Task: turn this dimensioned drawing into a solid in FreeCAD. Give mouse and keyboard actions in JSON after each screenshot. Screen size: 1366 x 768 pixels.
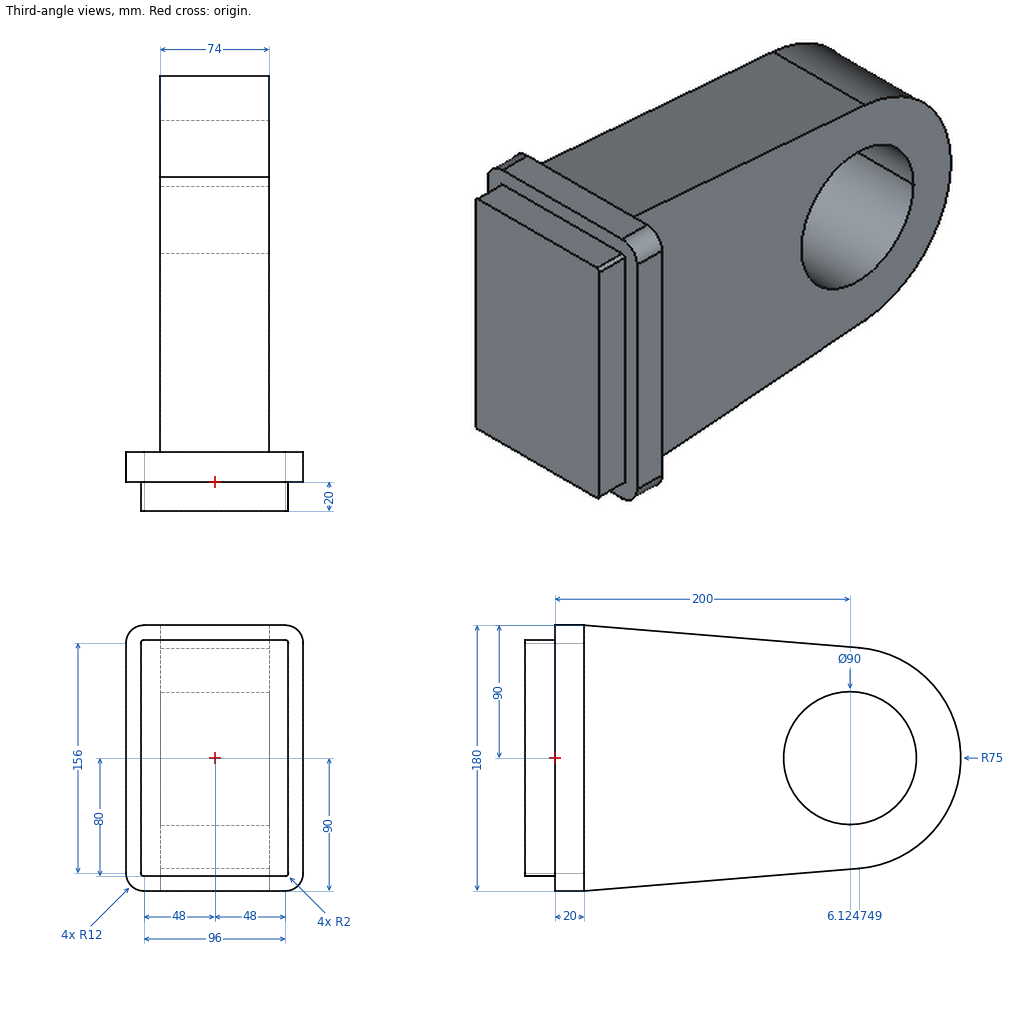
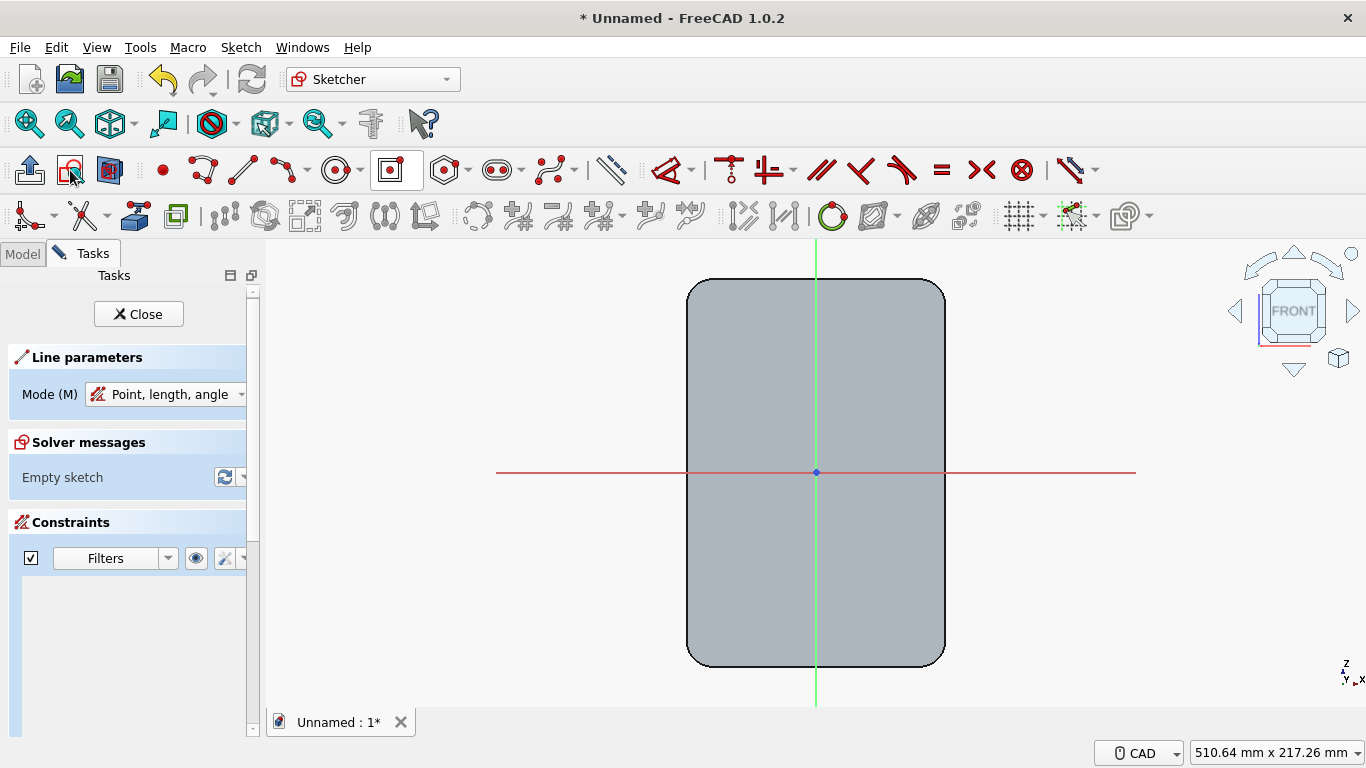
{"action": "left_click", "coordinate": [713, 645]}
{"action": "left_click", "coordinate": [919, 645]}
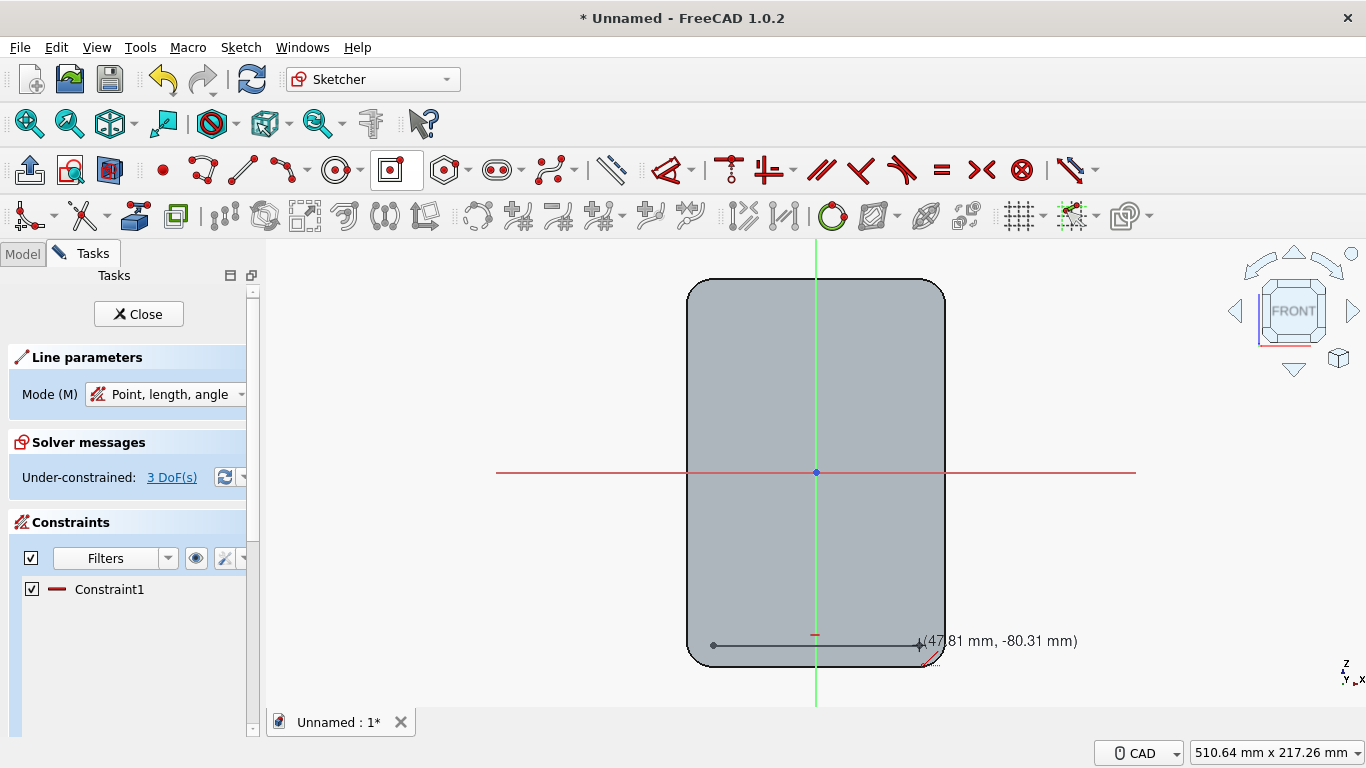
{"action": "scroll", "coordinate": [924, 641], "scroll_direction": "up", "scroll_amount": 5}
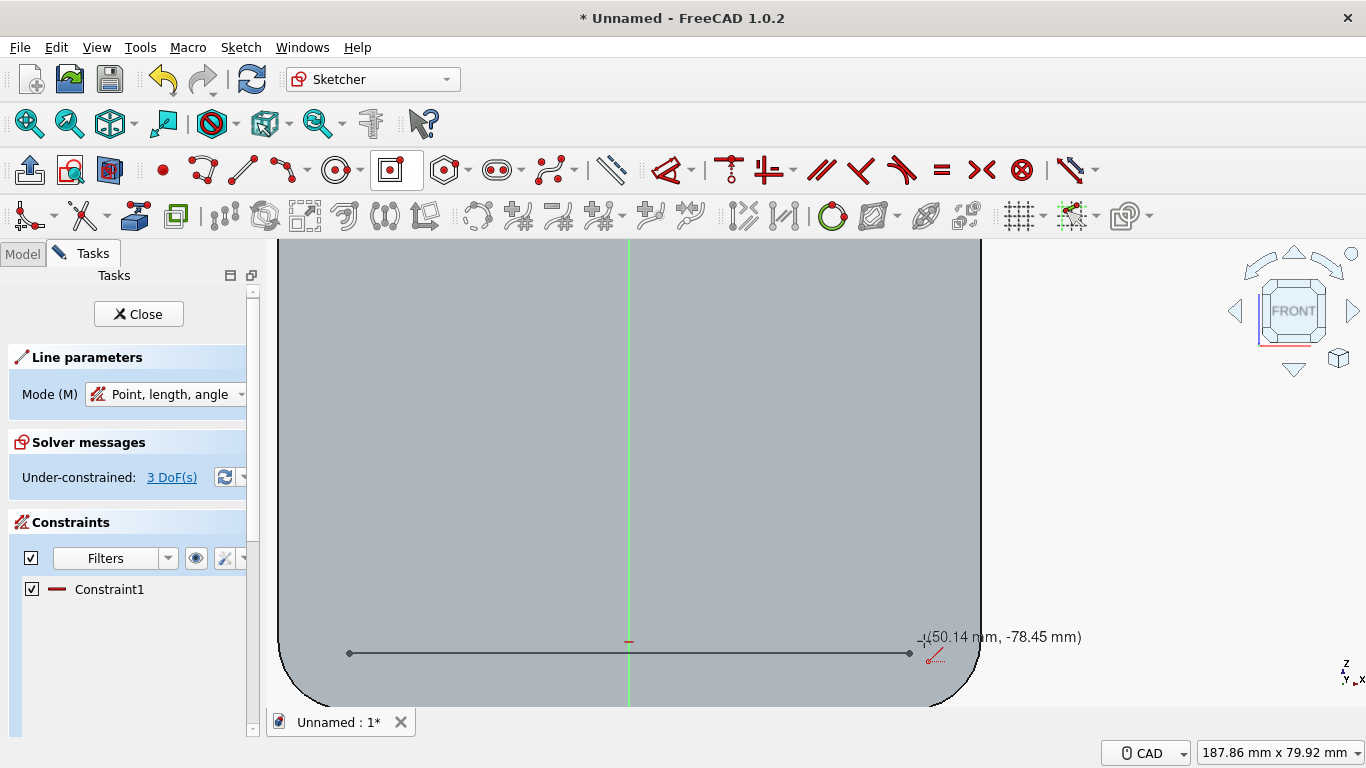
{"action": "left_click", "coordinate": [922, 640]}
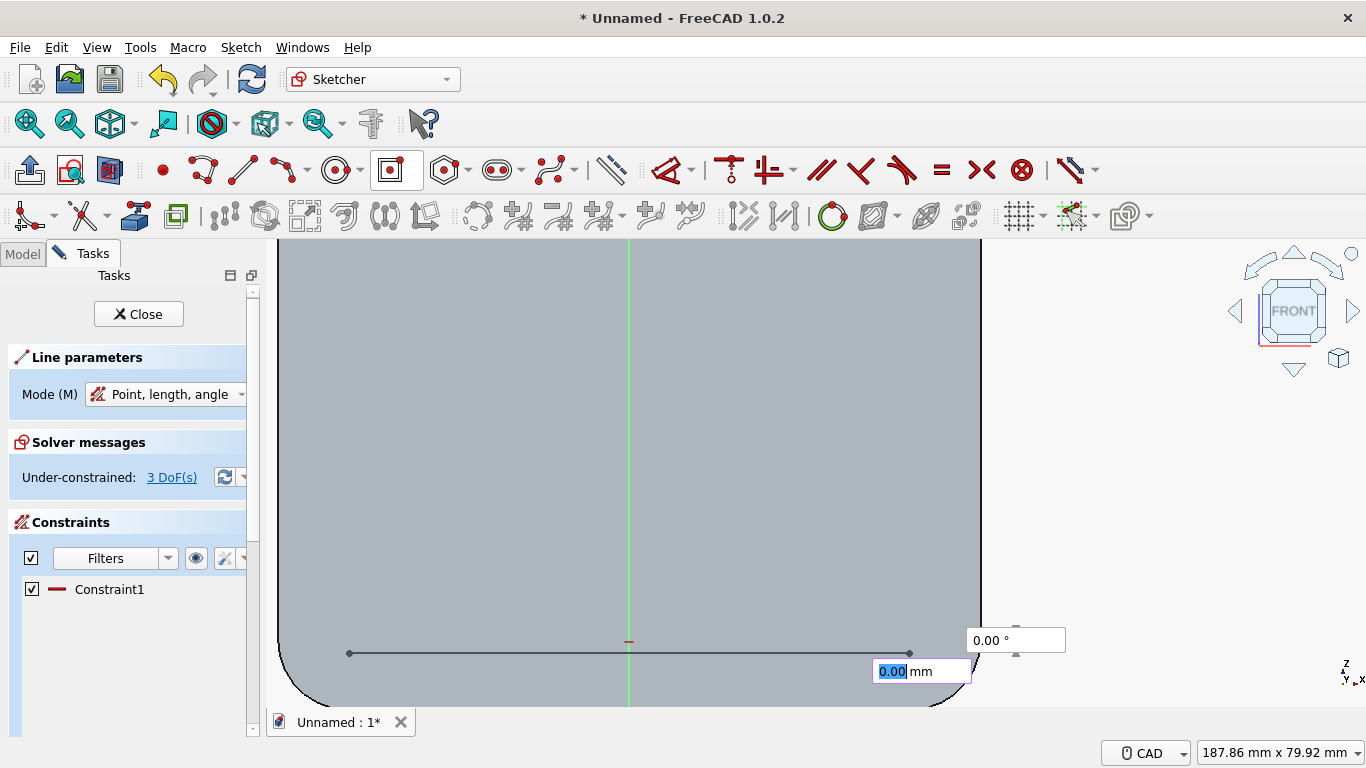
{"action": "scroll", "coordinate": [798, 598], "scroll_direction": "down", "scroll_amount": 6}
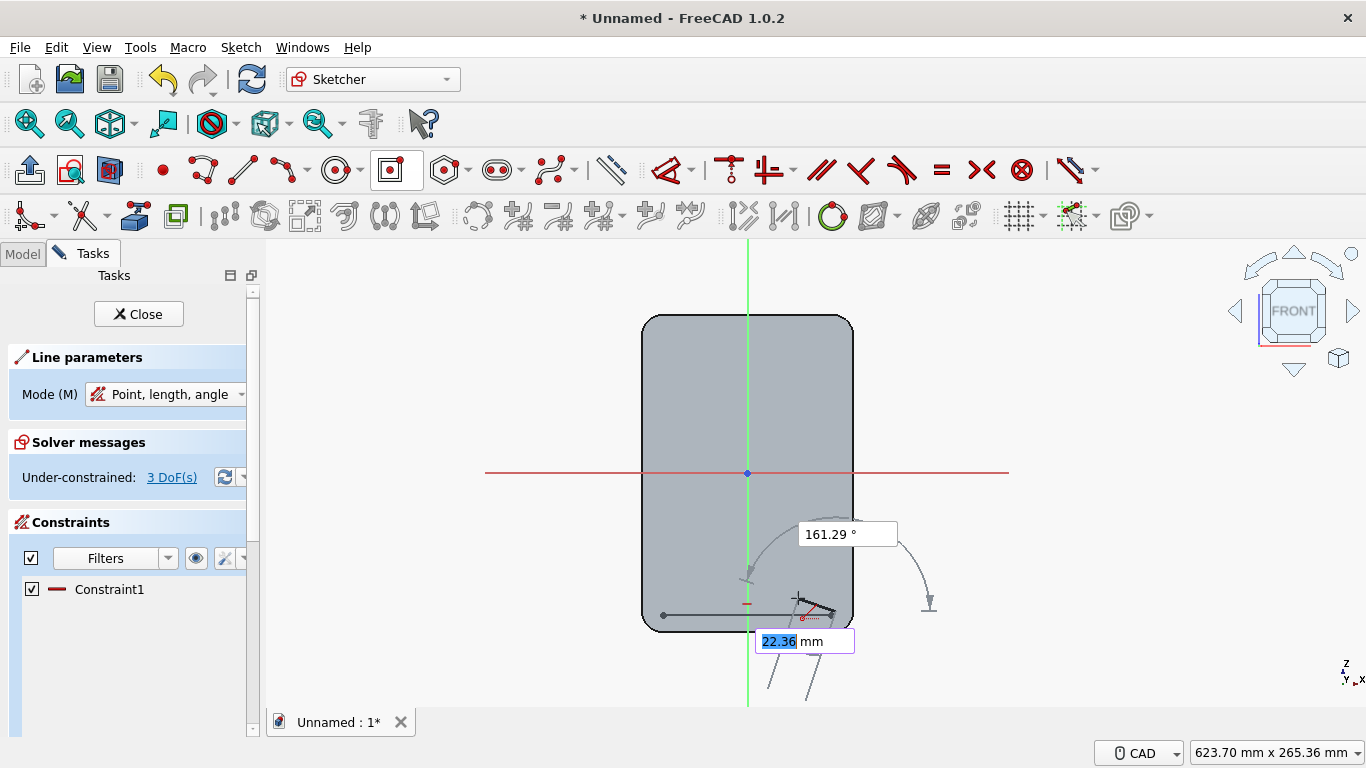
{"action": "left_click", "coordinate": [836, 336]}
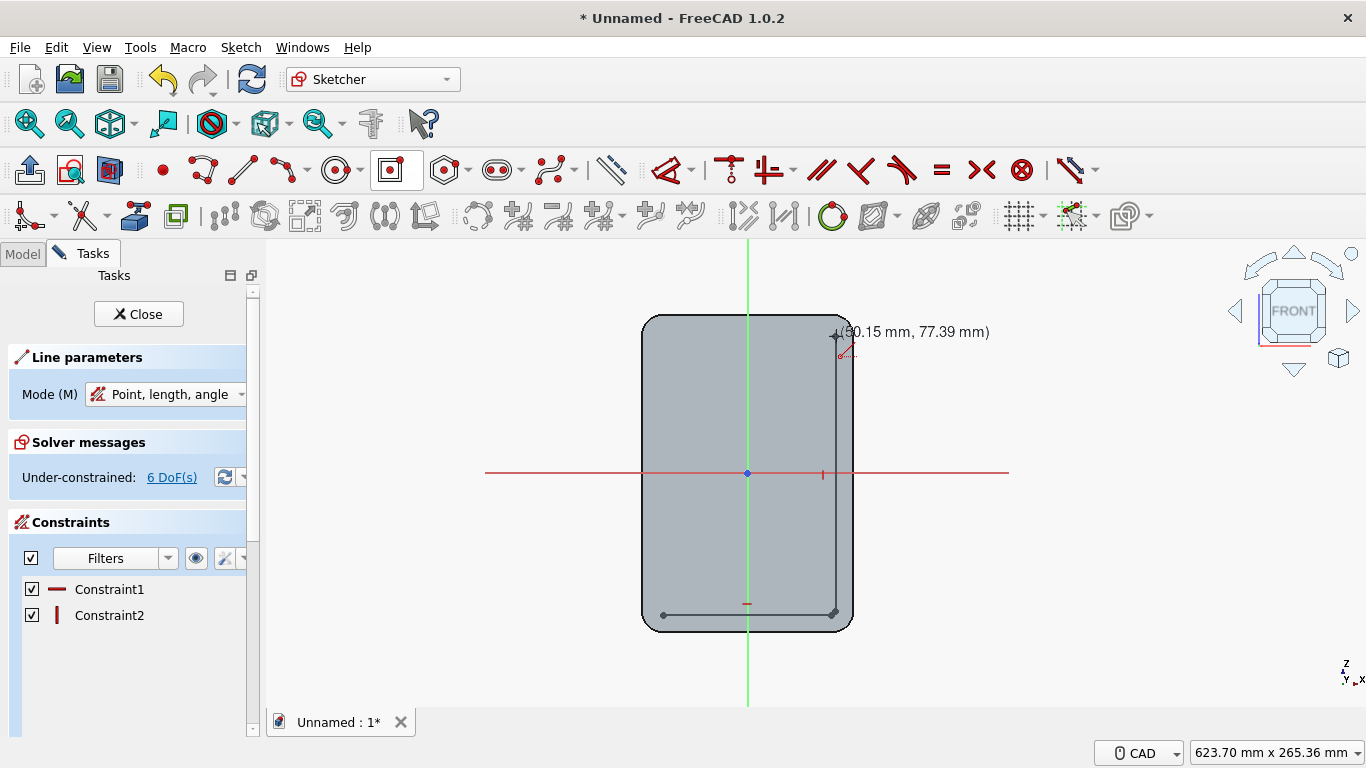
{"action": "scroll", "coordinate": [832, 332], "scroll_direction": "up", "scroll_amount": 6}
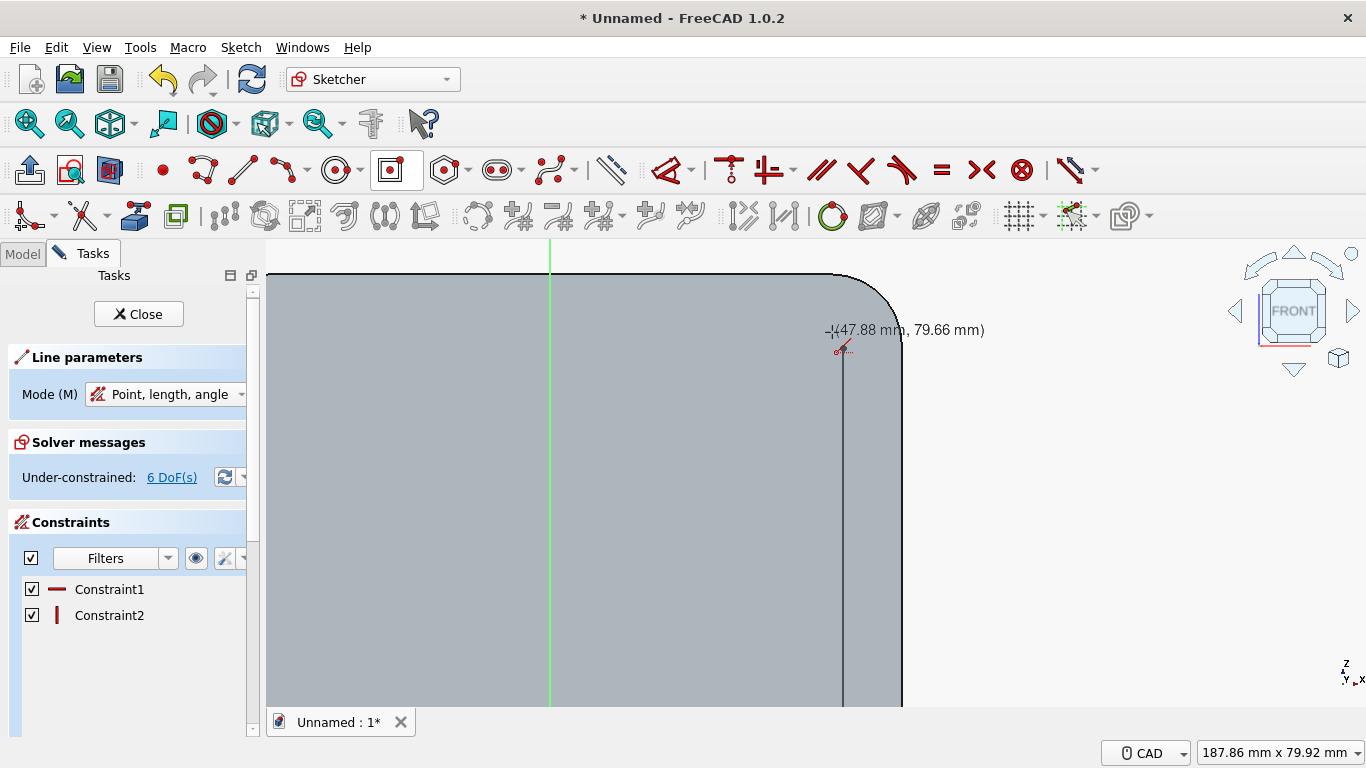
{"action": "left_click", "coordinate": [832, 333]}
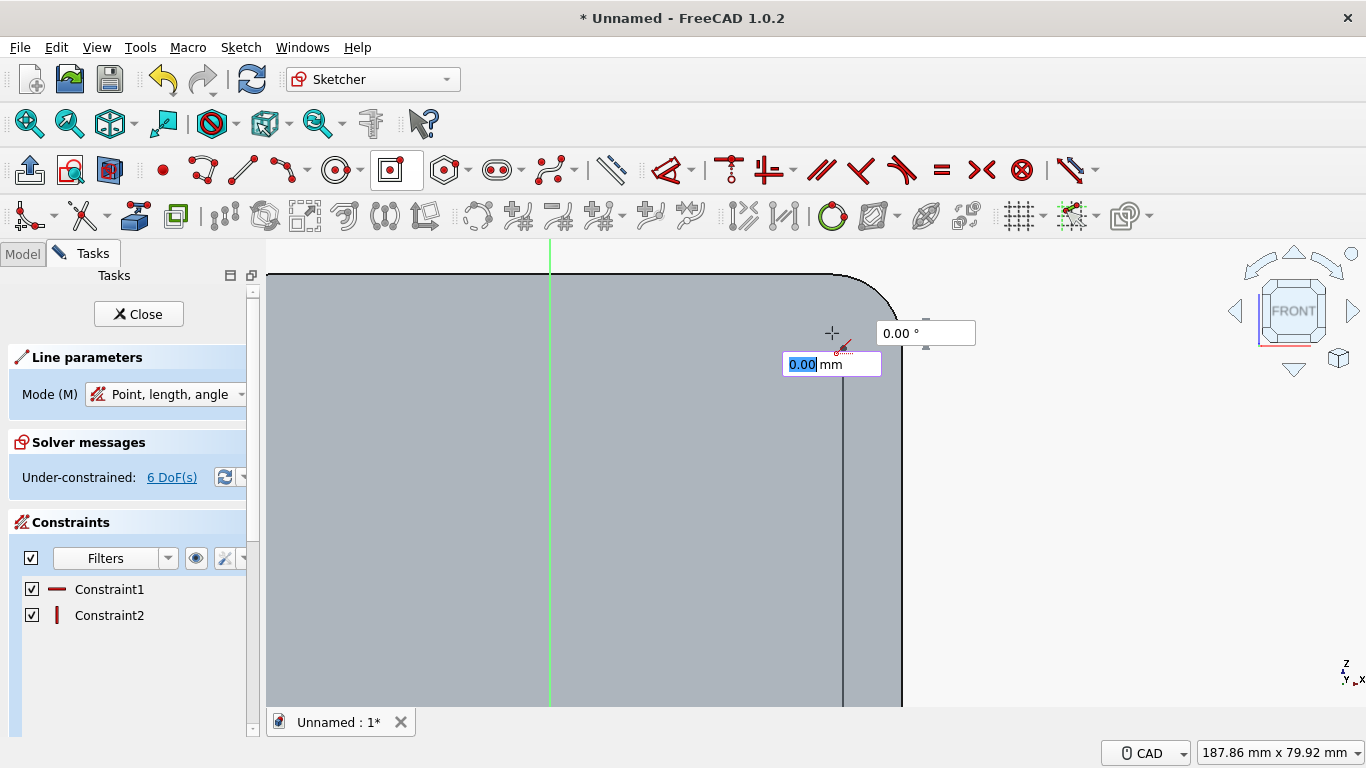
{"action": "scroll", "coordinate": [832, 331], "scroll_direction": "down", "scroll_amount": 6}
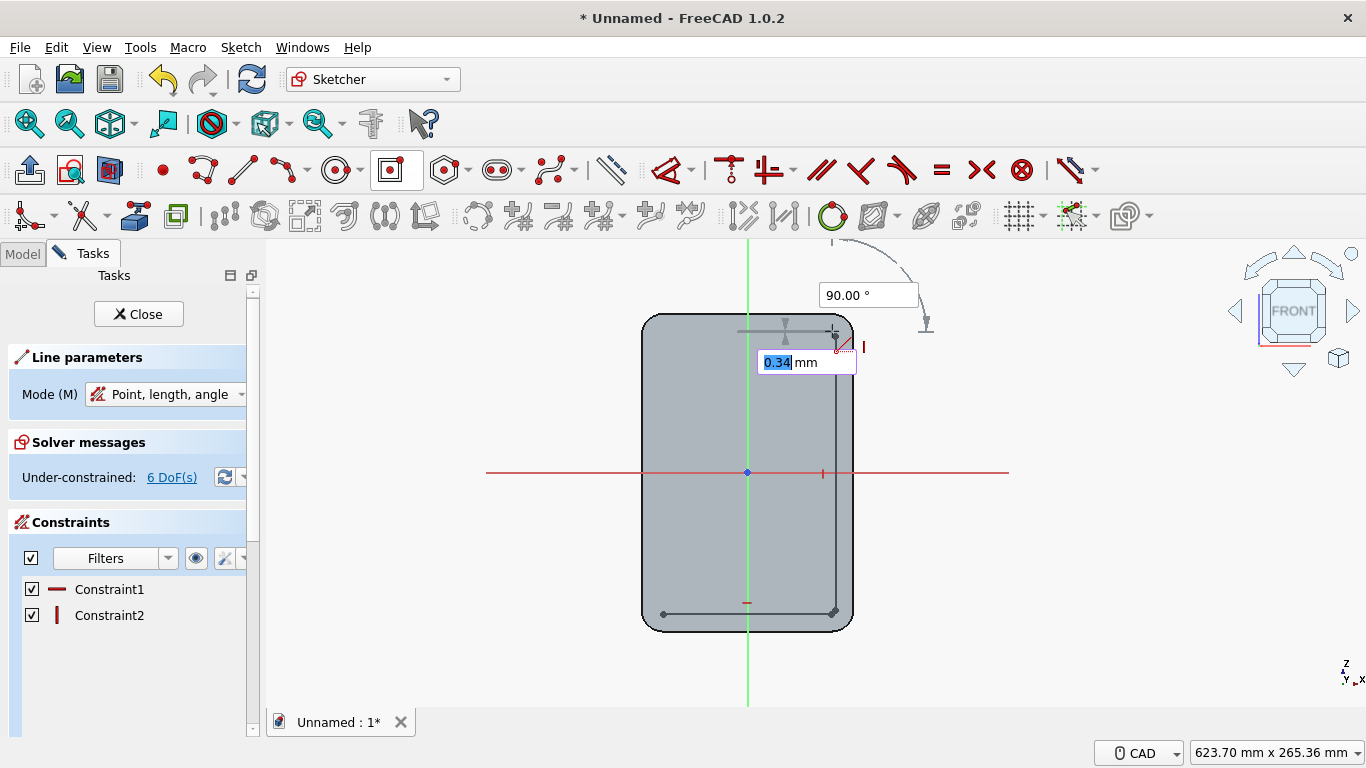
{"action": "left_click", "coordinate": [663, 332]}